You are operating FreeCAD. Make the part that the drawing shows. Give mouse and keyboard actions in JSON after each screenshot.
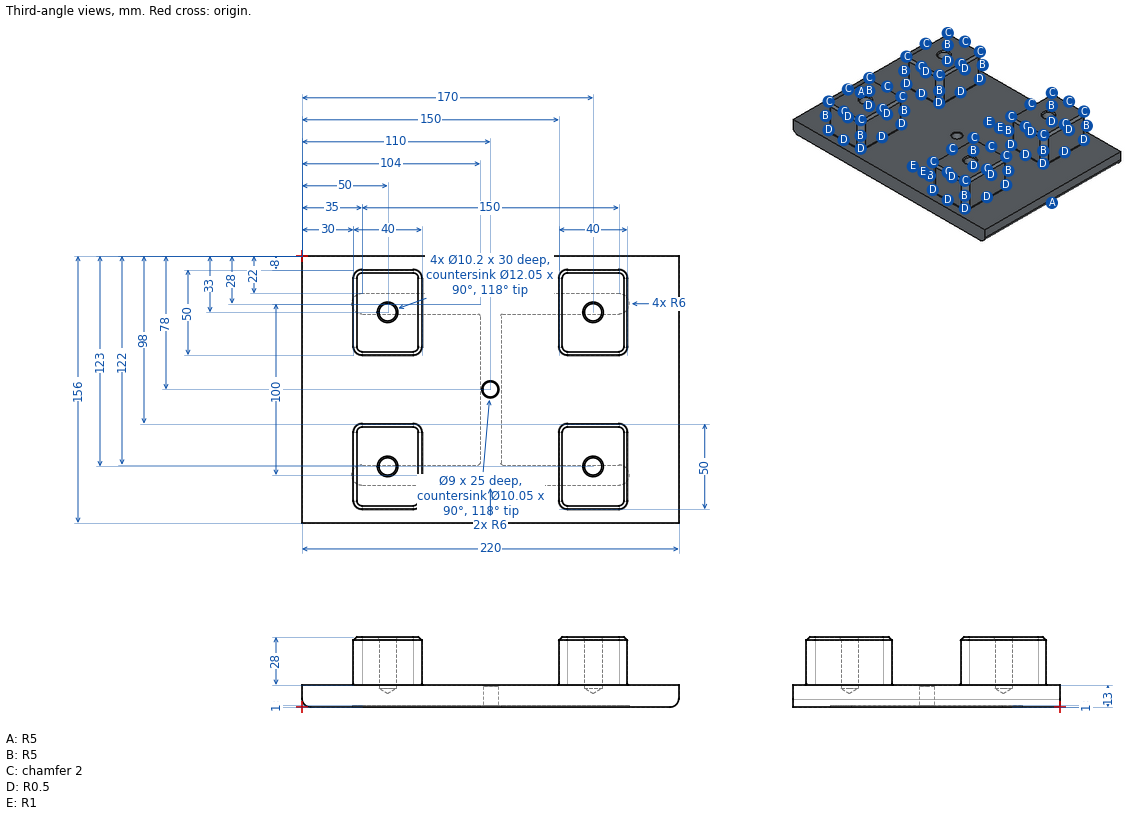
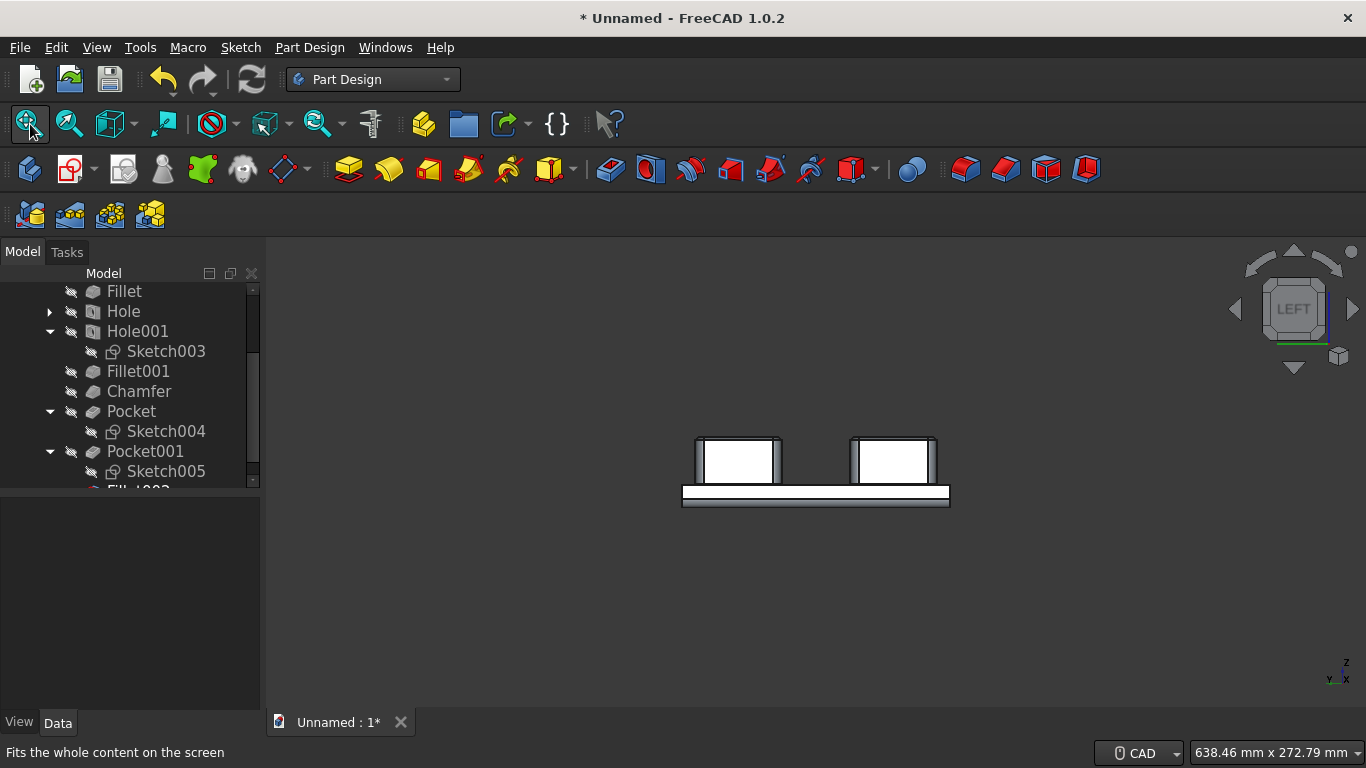
{"action": "left_click", "coordinate": [30, 124]}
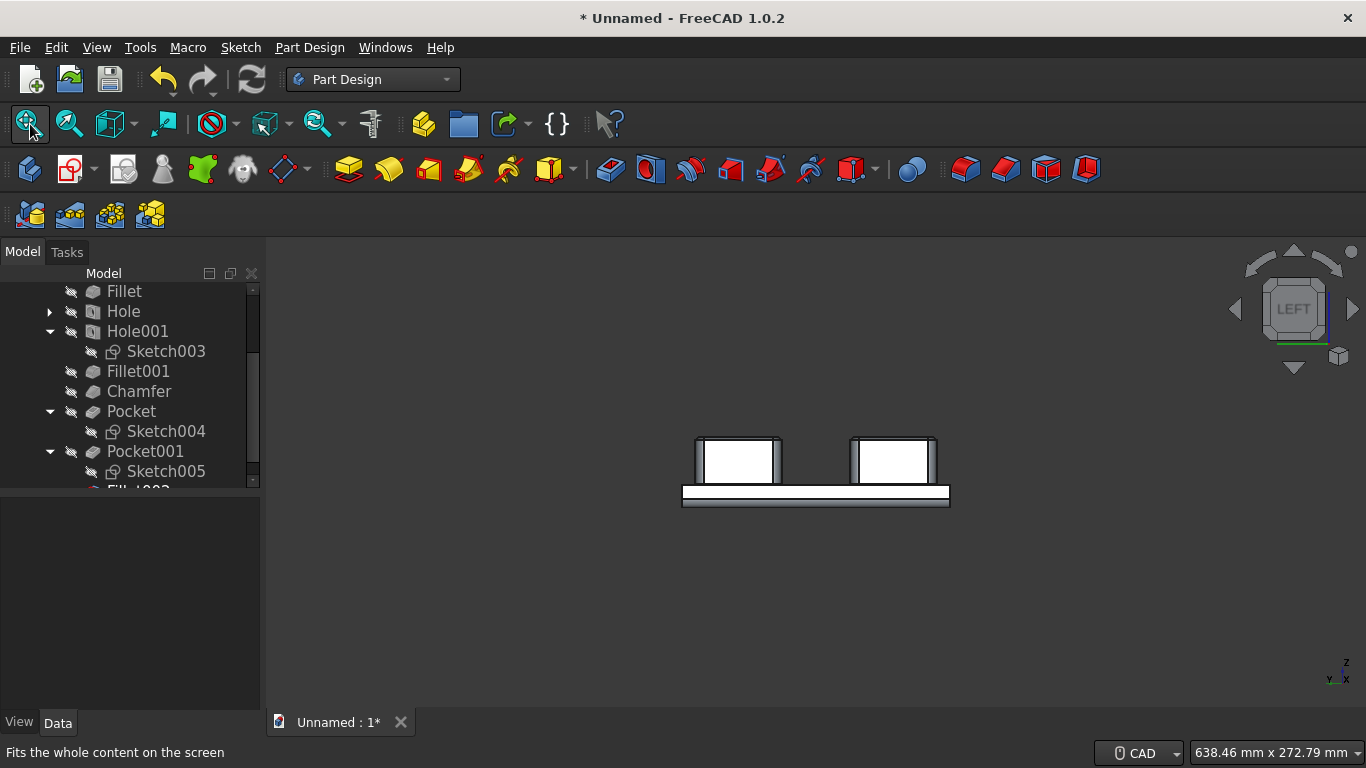
{"action": "scroll", "coordinate": [892, 505], "scroll_direction": "up", "scroll_amount": 15}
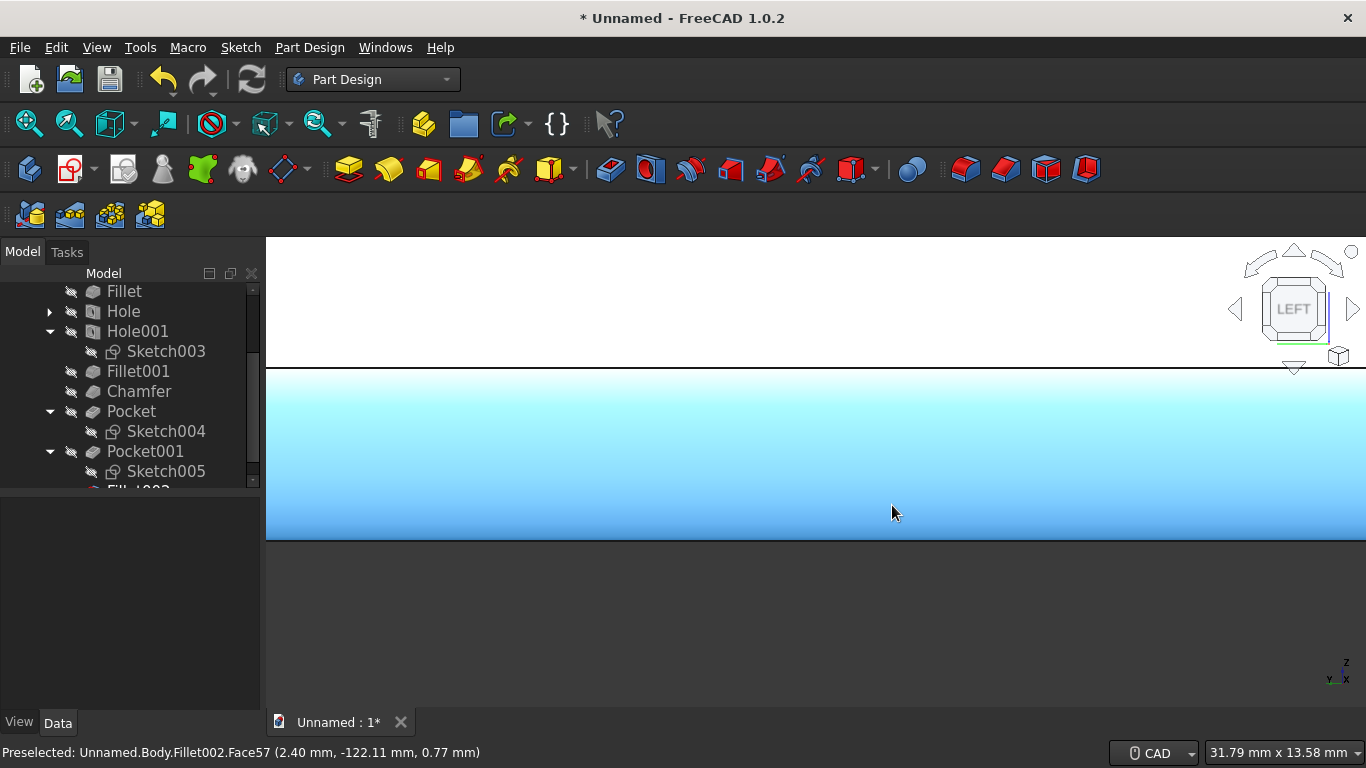
{"action": "key", "text": "v f"}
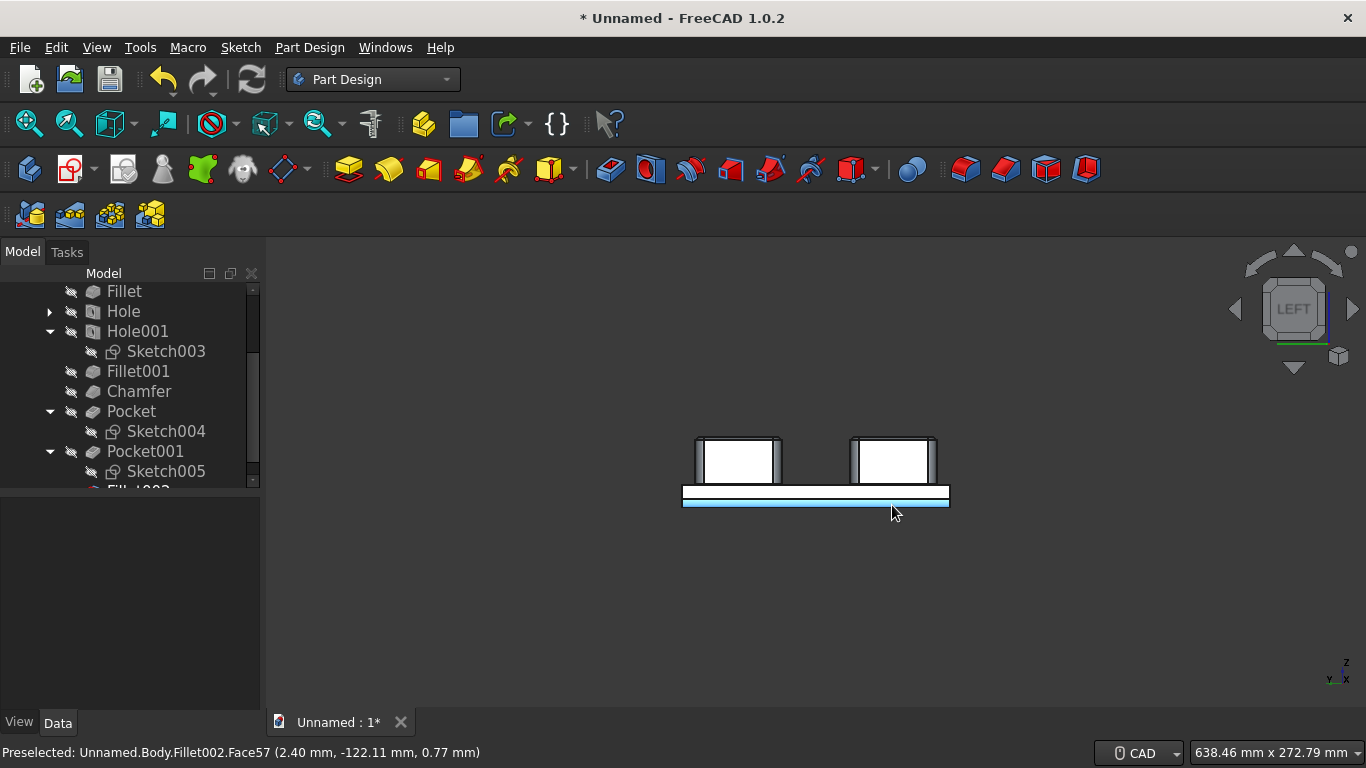
{"action": "key", "text": "v 3"}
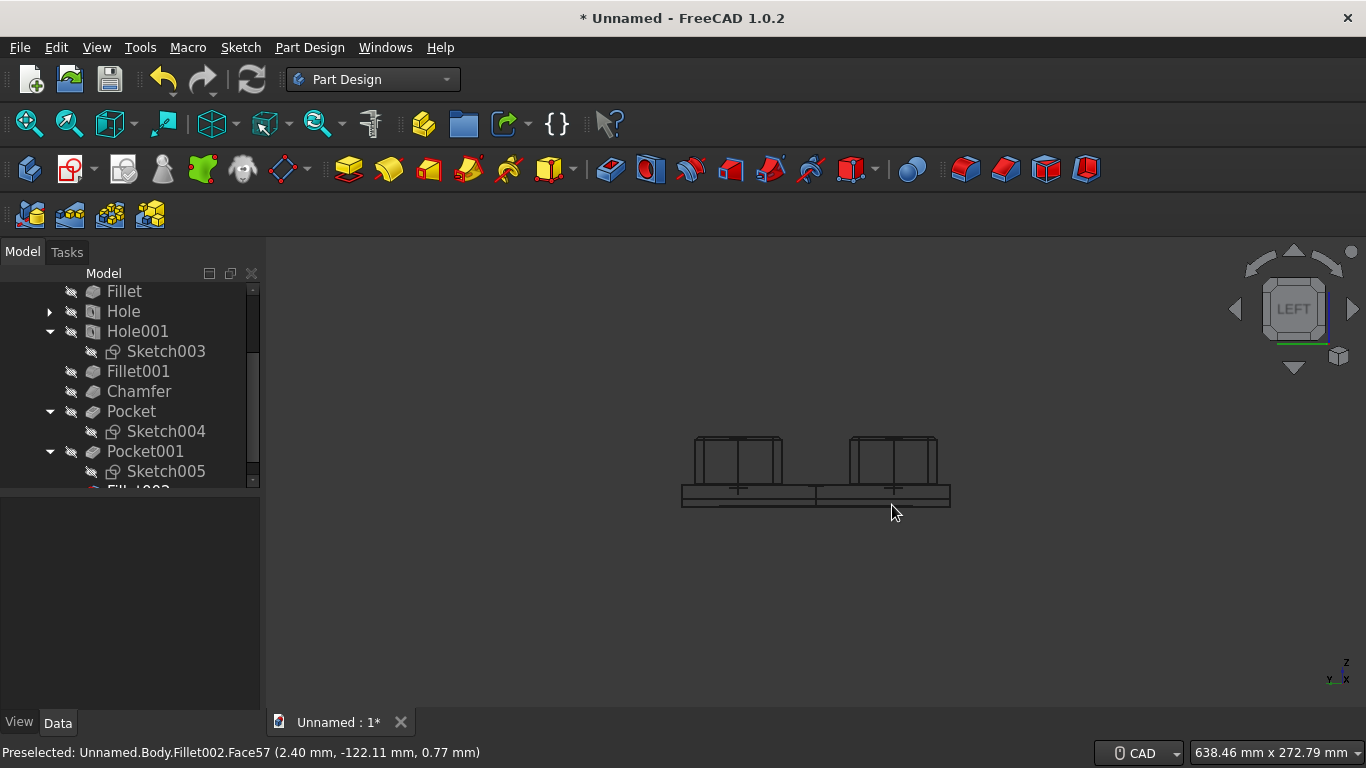
{"action": "key", "text": "0"}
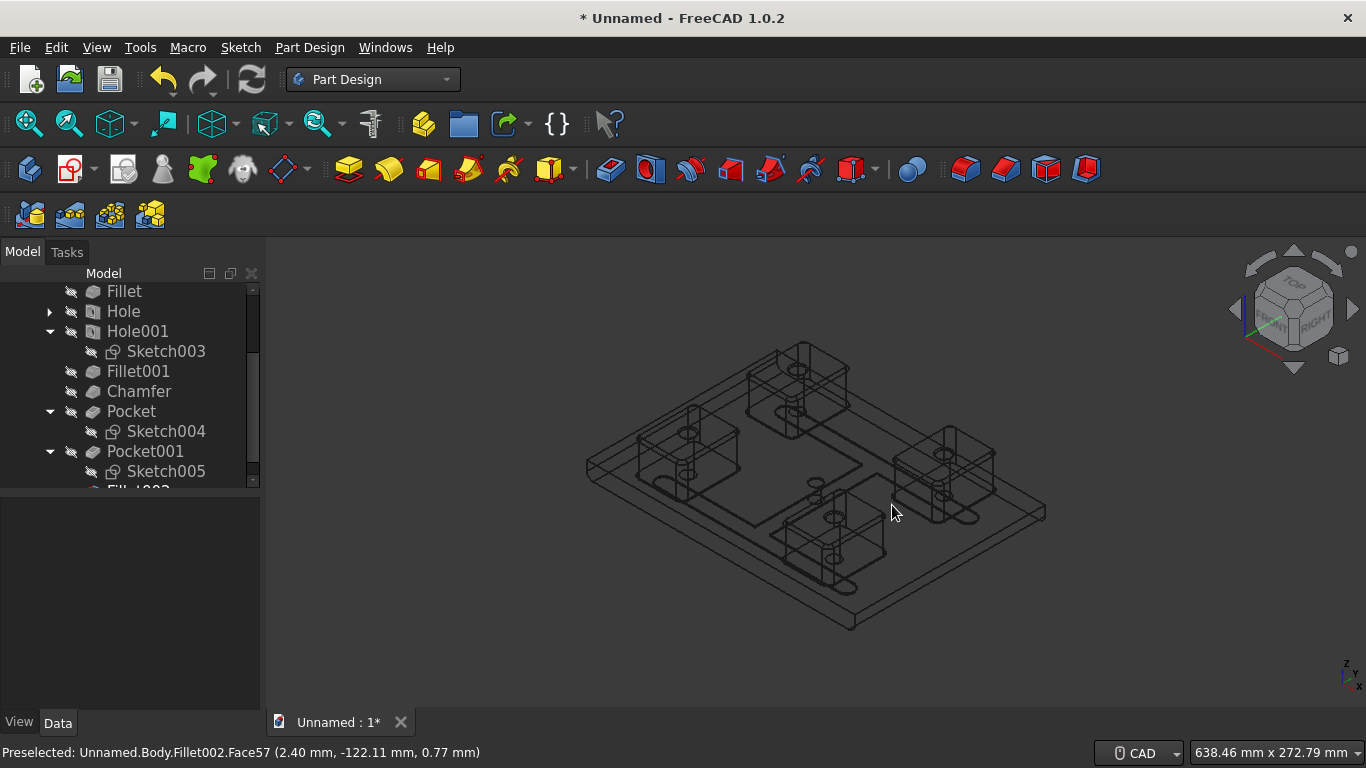
{"action": "scroll", "coordinate": [755, 526], "scroll_direction": "up", "scroll_amount": 15}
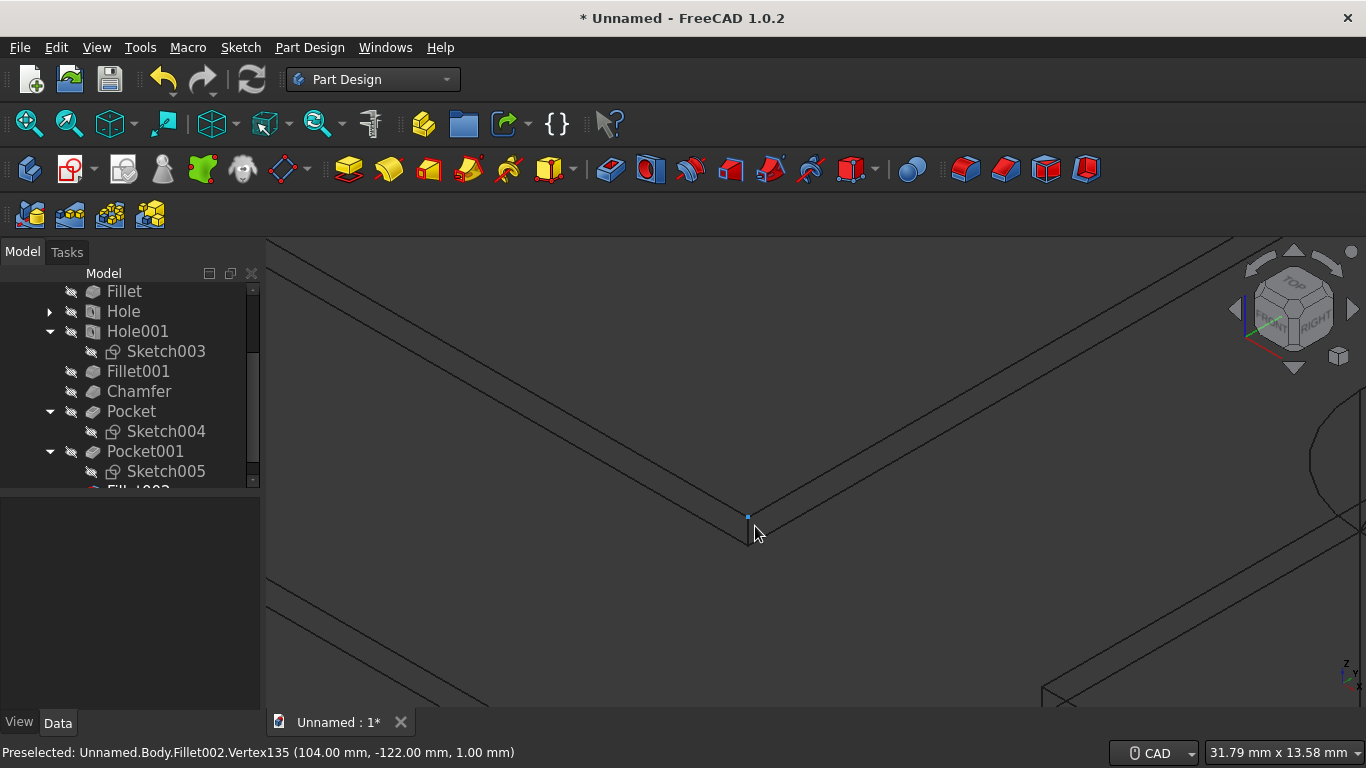
{"action": "left_click", "coordinate": [748, 531]}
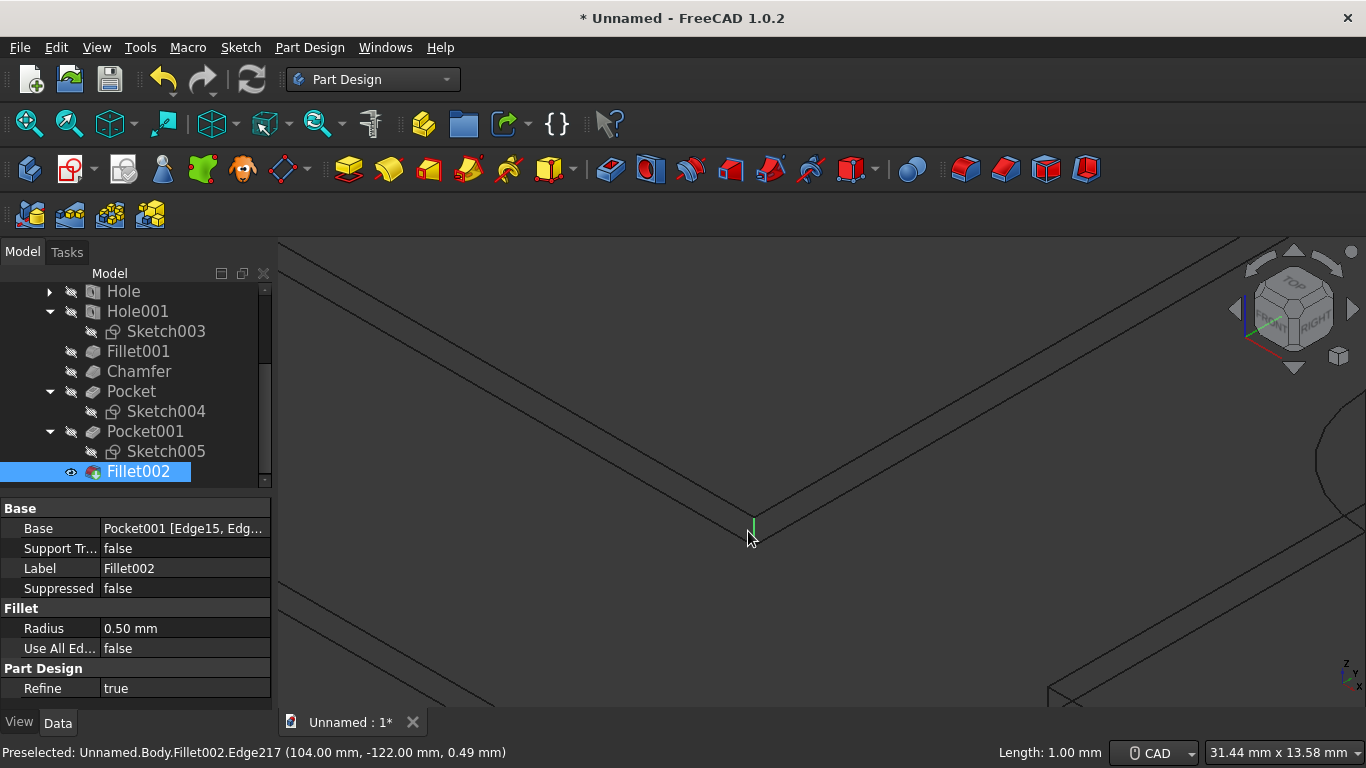
{"action": "key", "text": "v f"}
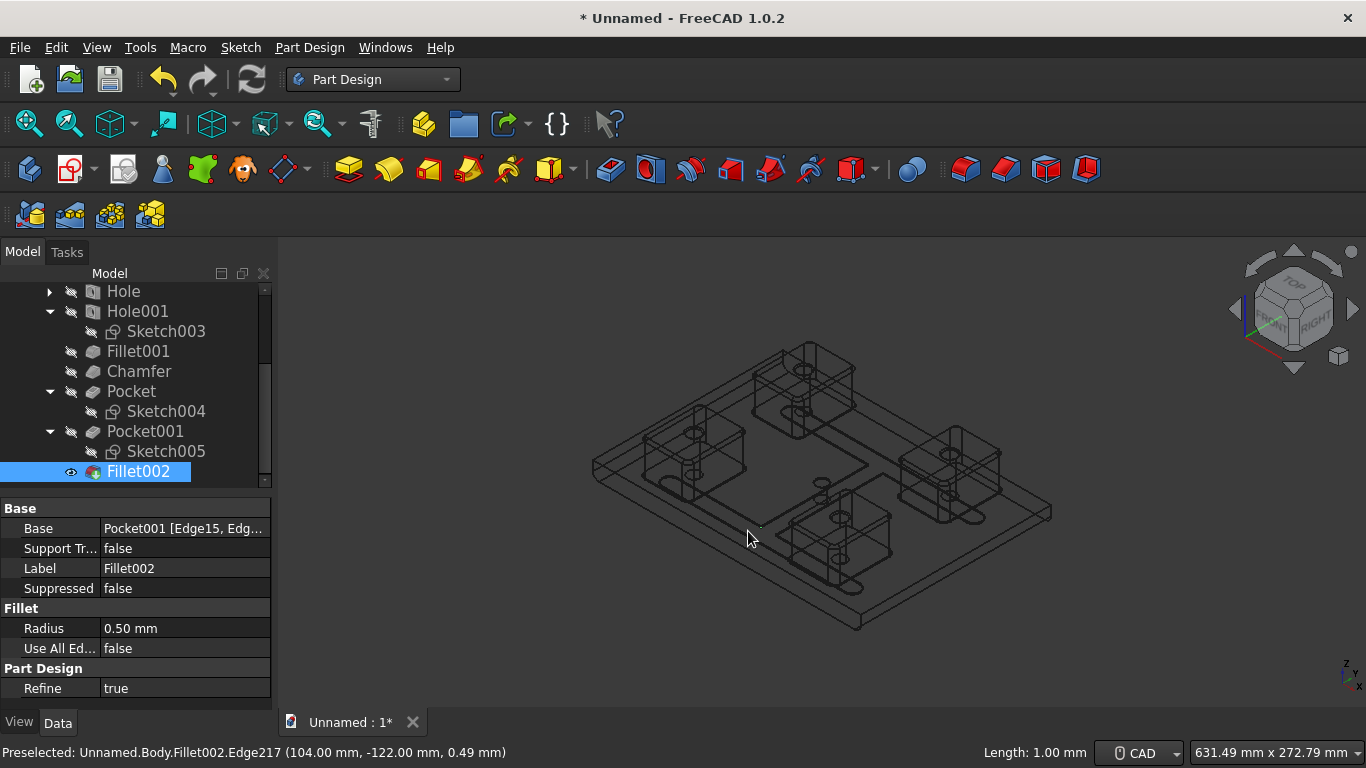
{"action": "key", "text": "2"}